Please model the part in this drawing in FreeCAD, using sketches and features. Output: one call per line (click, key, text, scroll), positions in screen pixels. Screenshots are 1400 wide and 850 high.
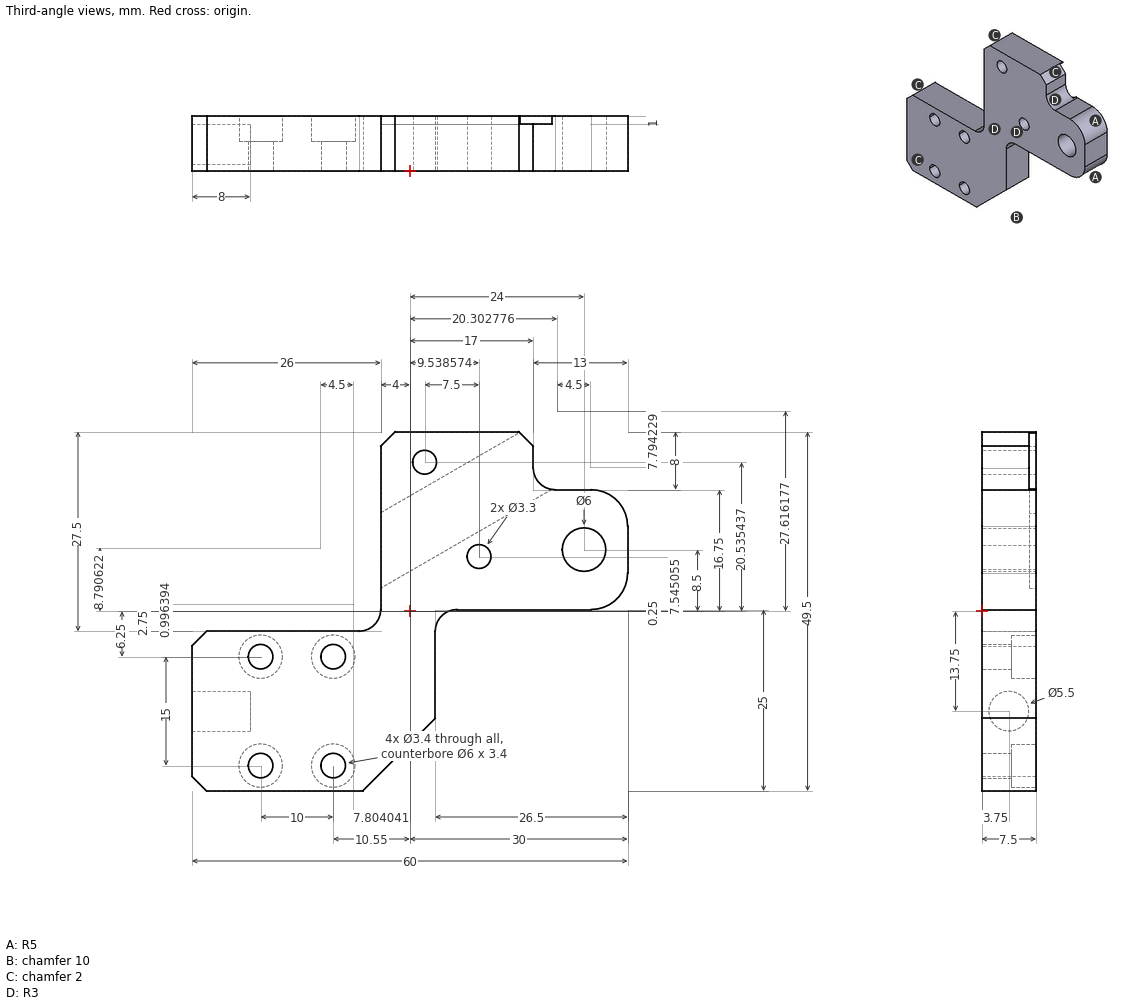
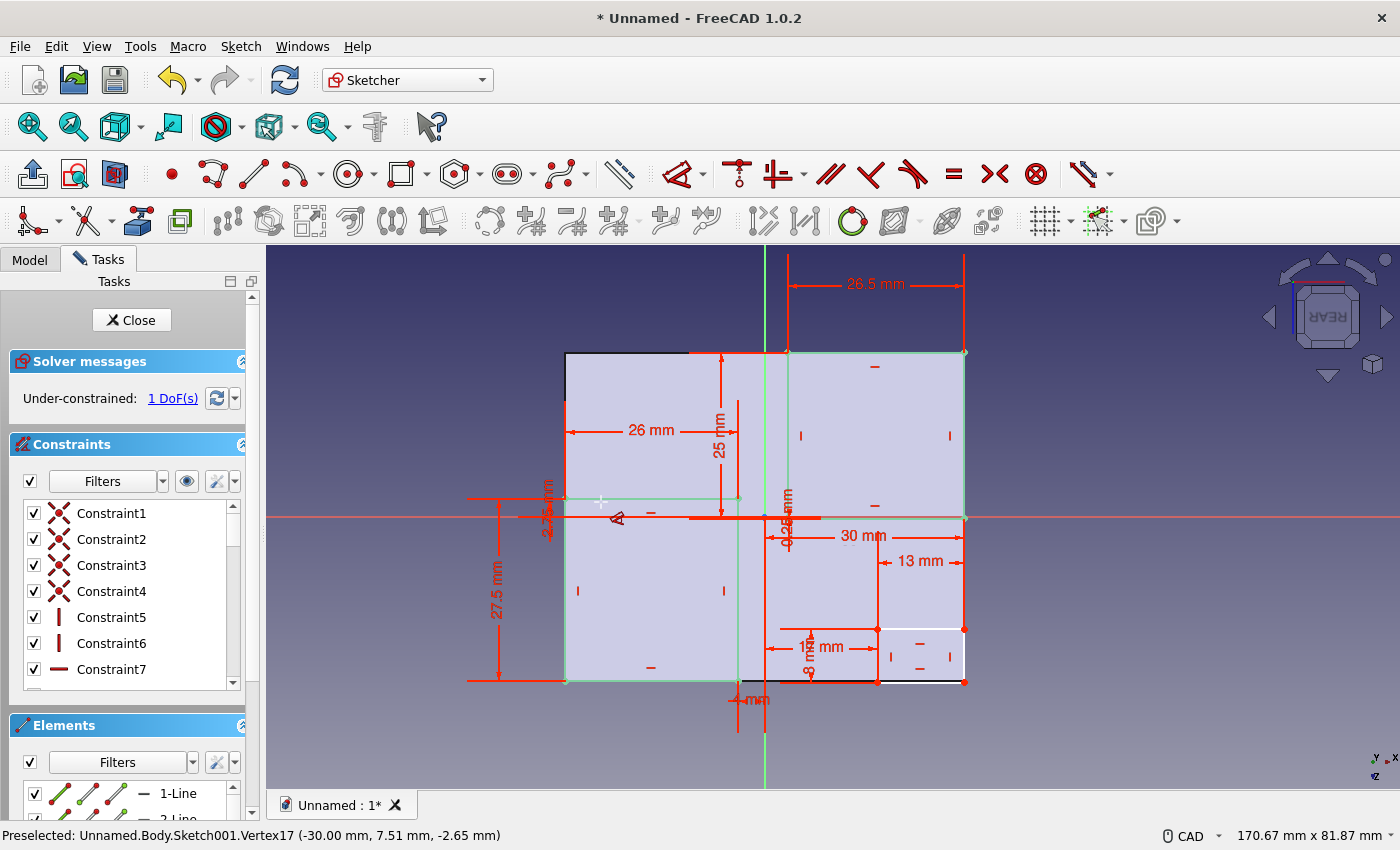
click(878, 629)
click(912, 573)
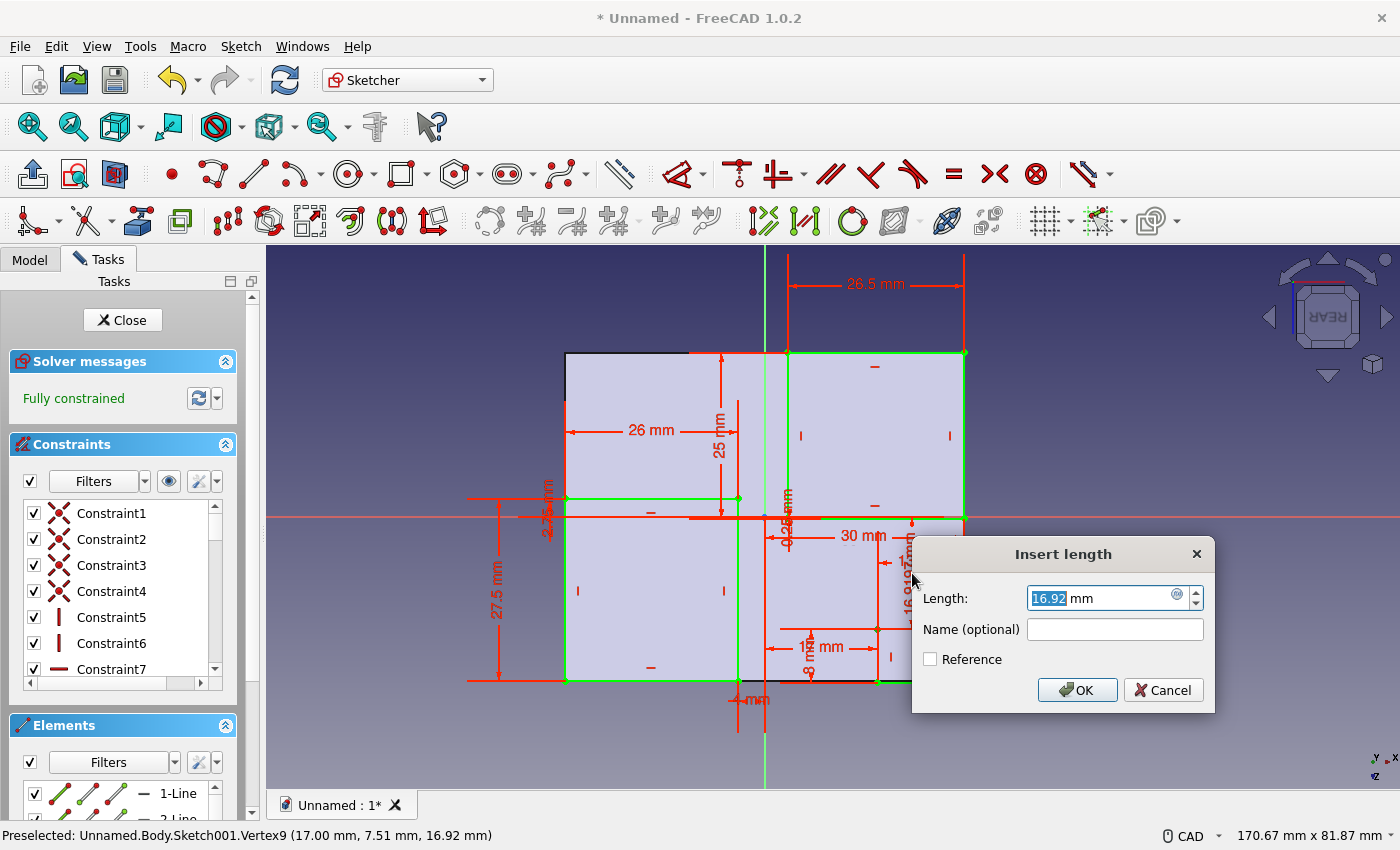
text(16.75)
key(Return)
key(Escape)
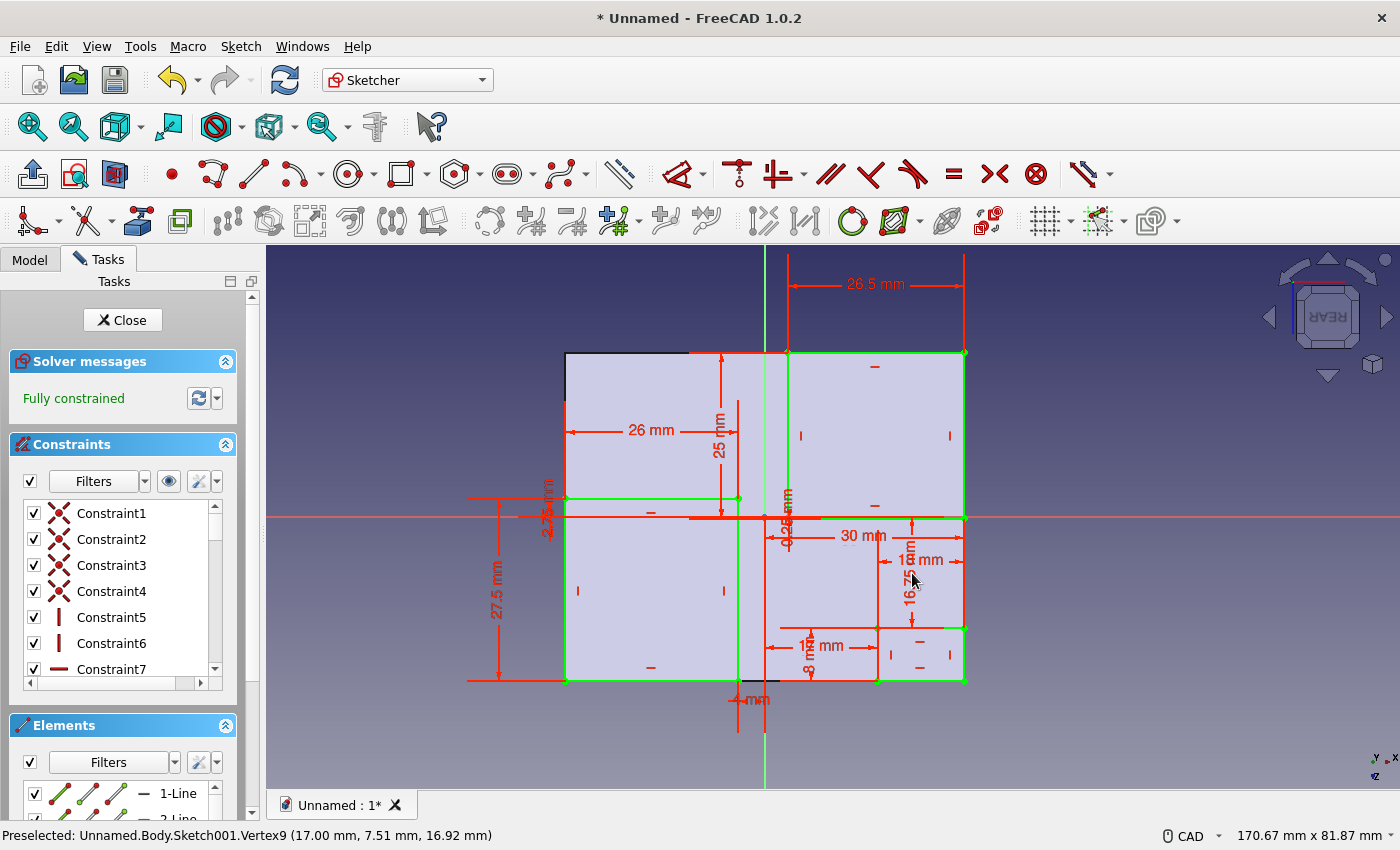
click(123, 320)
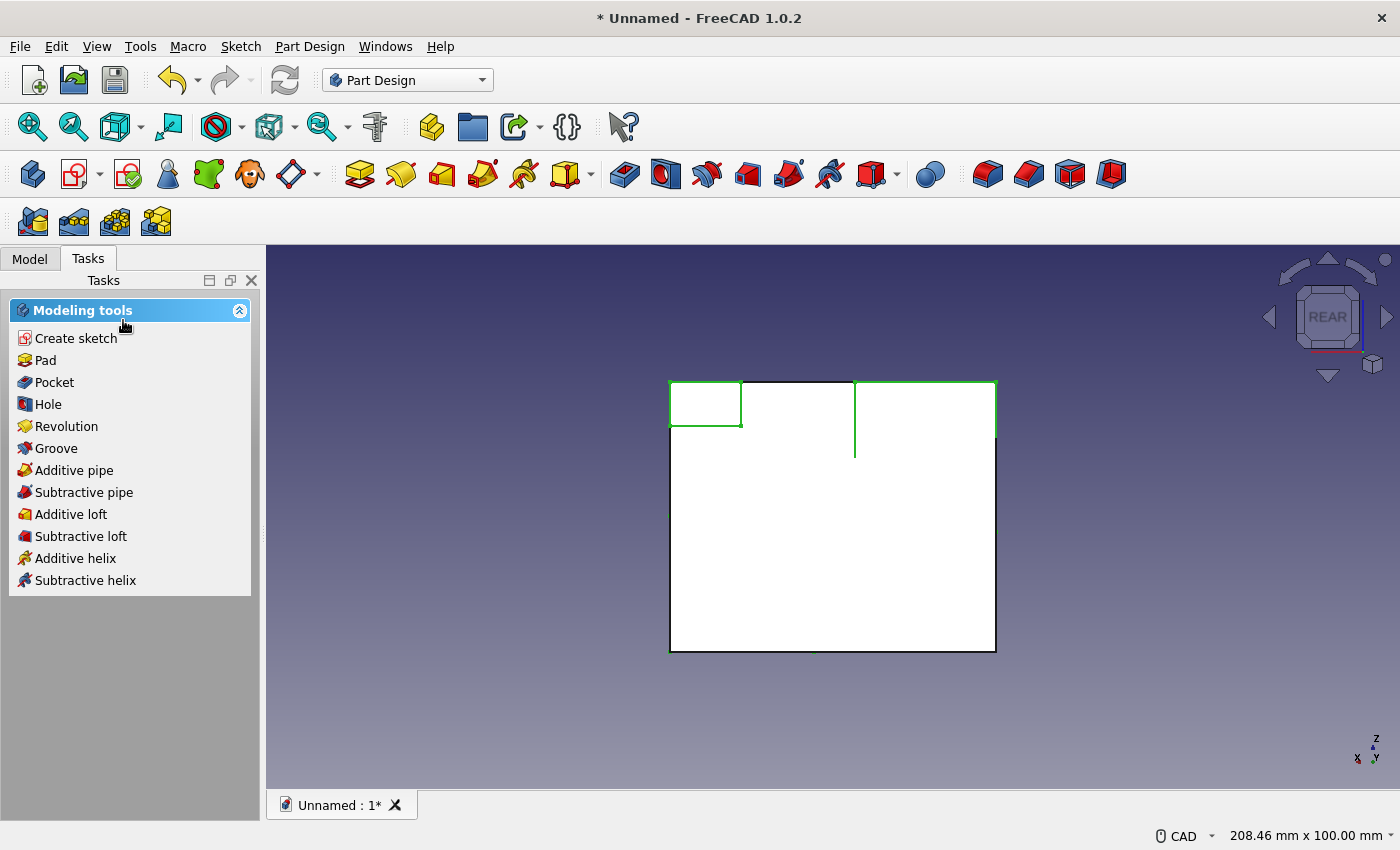
click(625, 174)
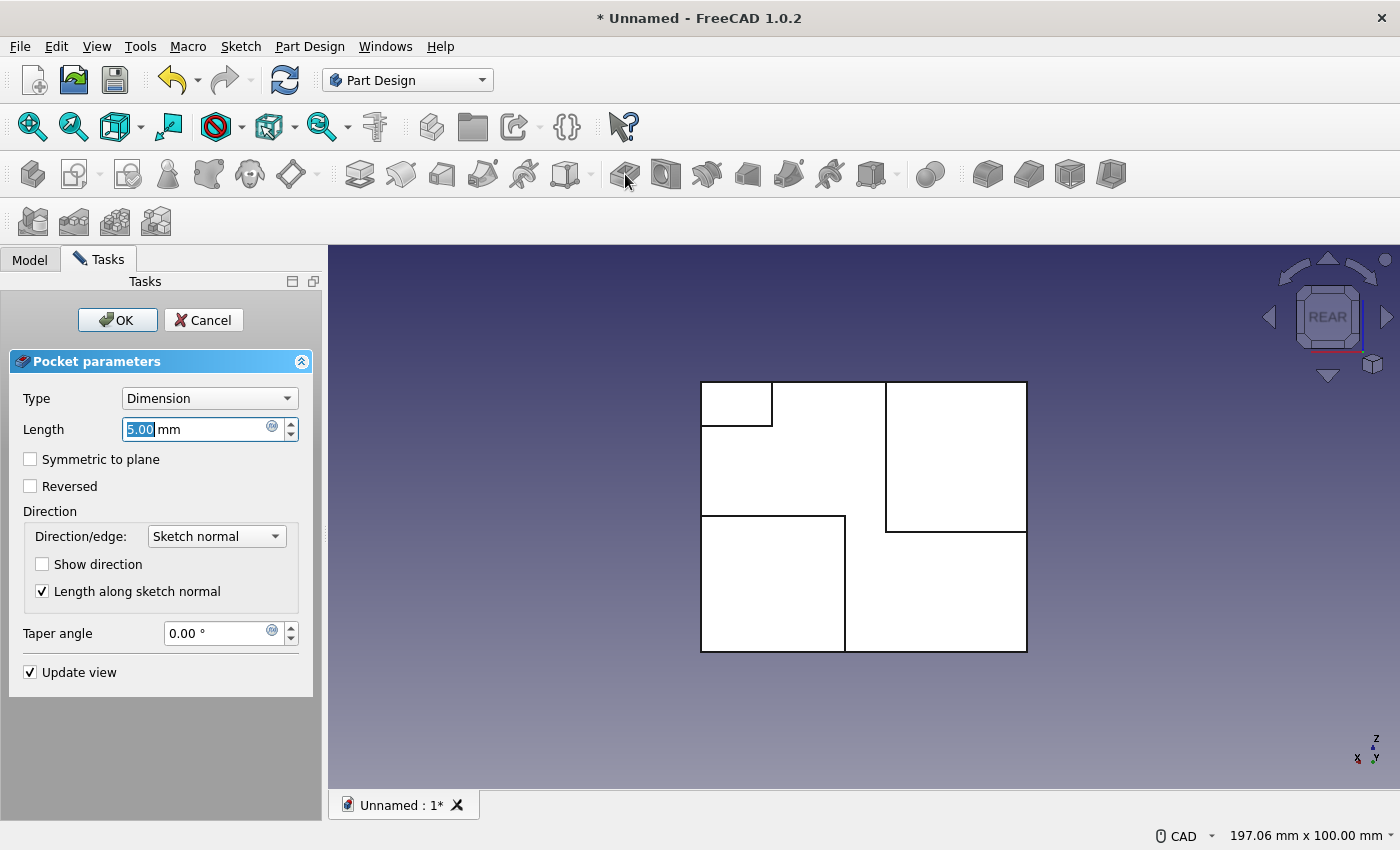
click(210, 398)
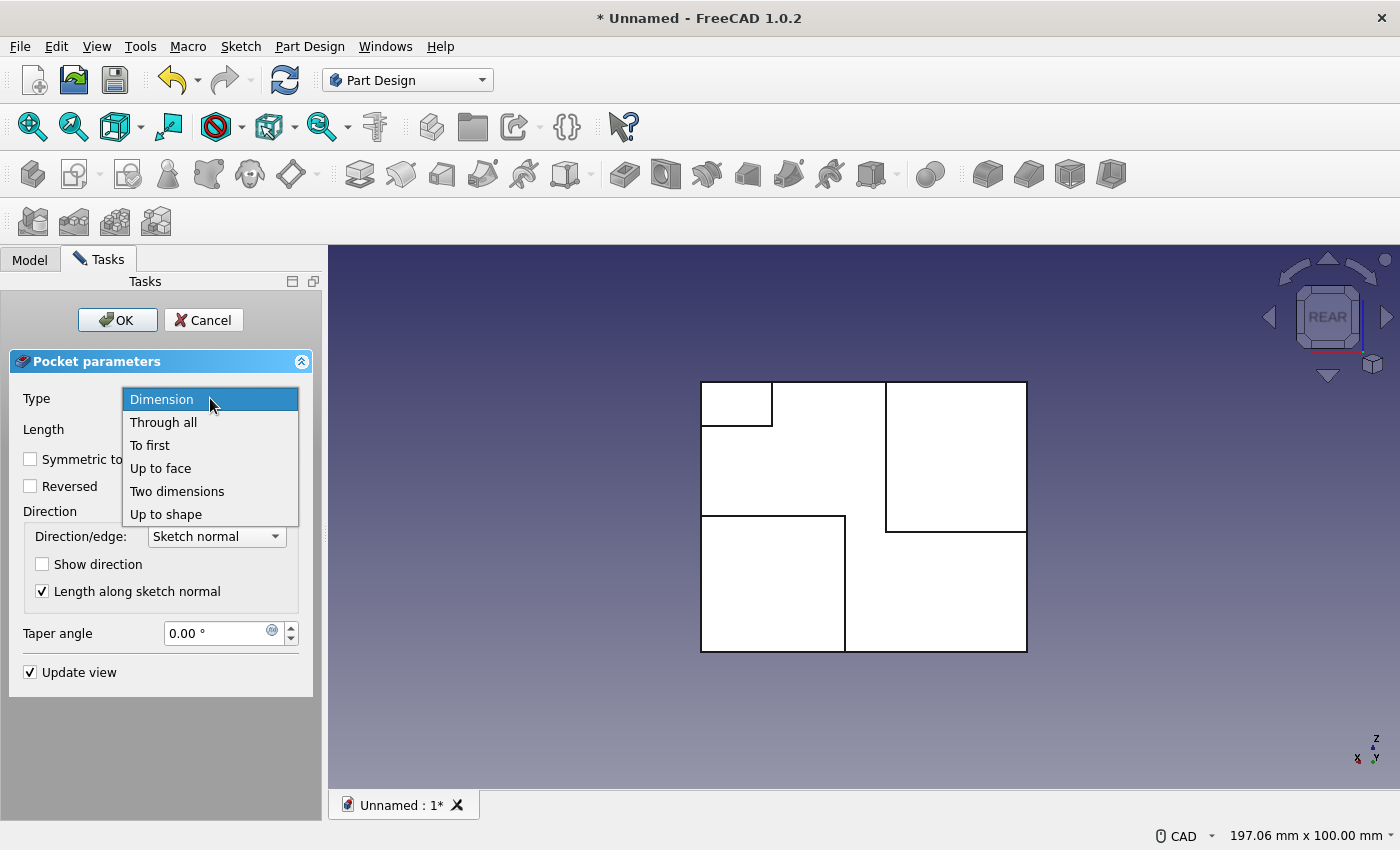
click(208, 422)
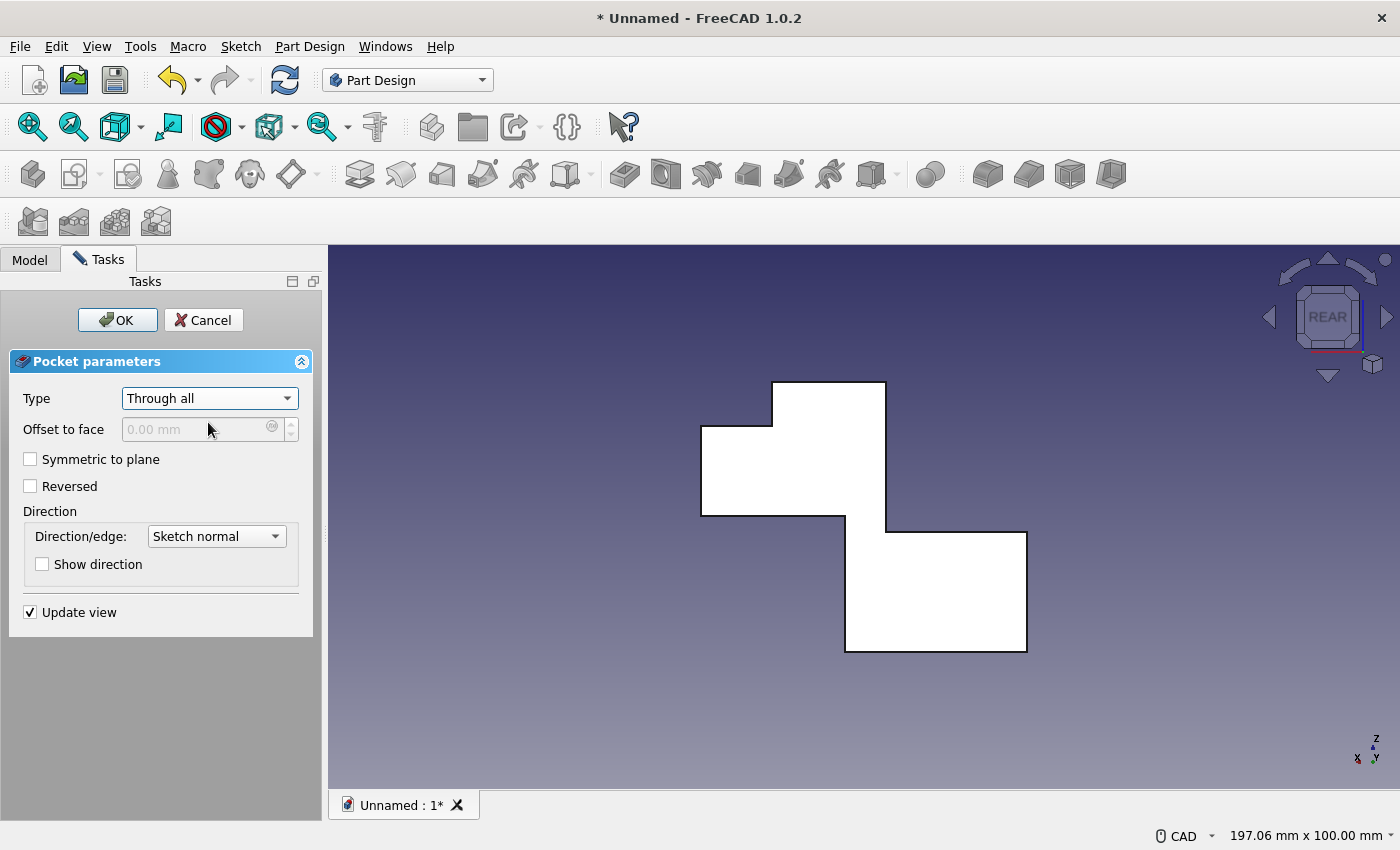
click(118, 320)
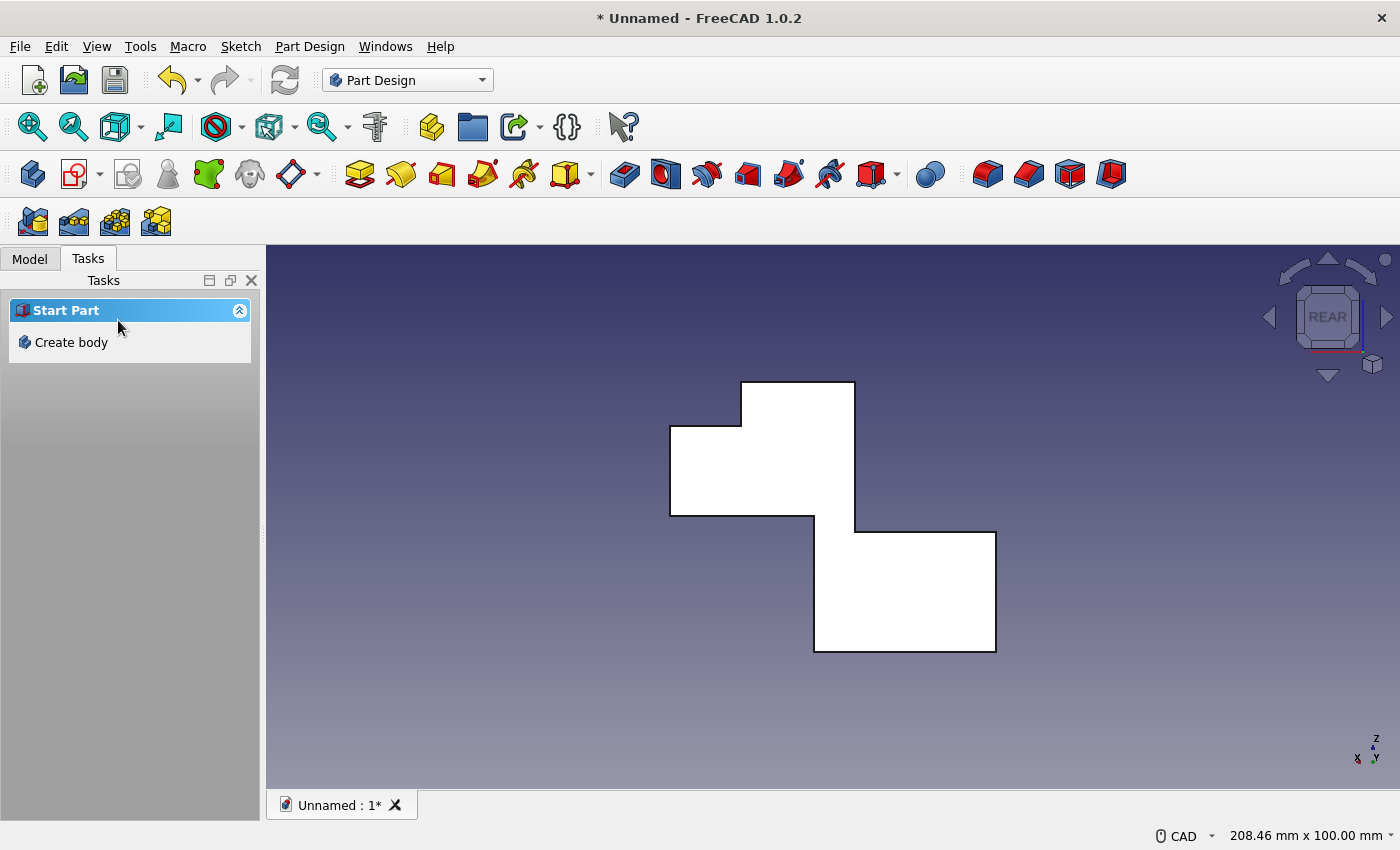
click(880, 593)